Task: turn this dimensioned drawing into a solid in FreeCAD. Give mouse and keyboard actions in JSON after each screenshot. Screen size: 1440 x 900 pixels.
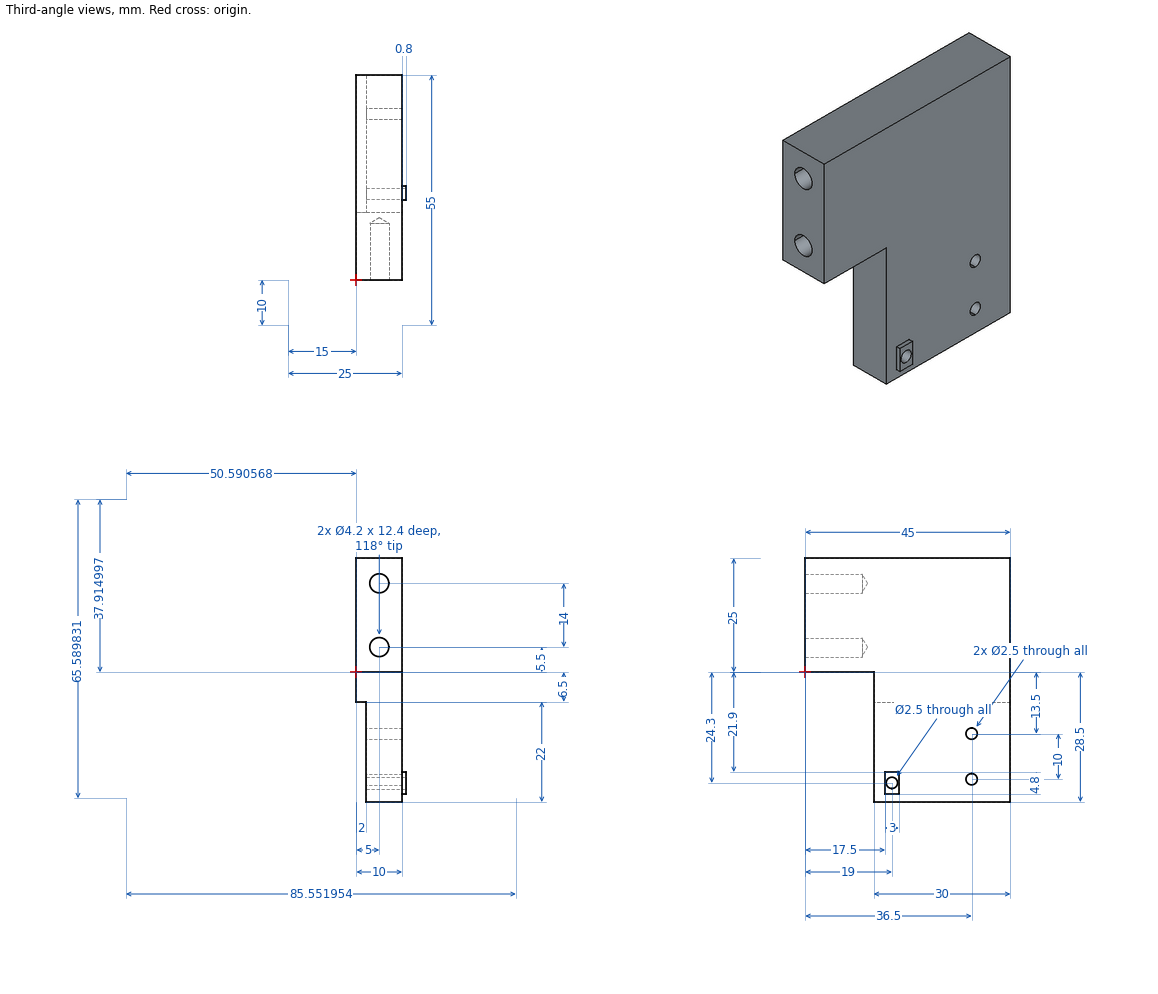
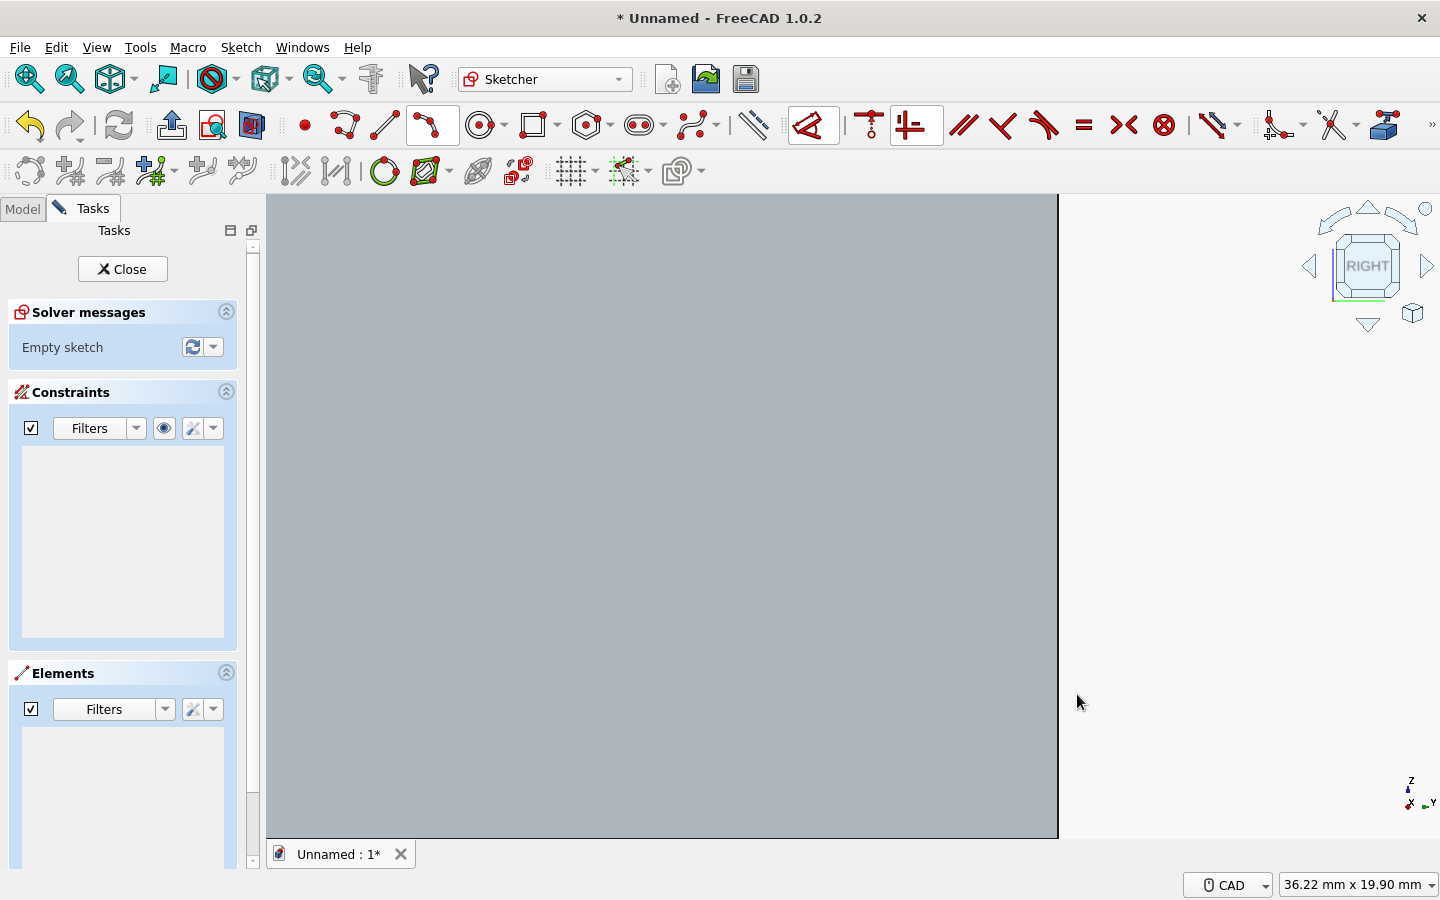
{"action": "left_click", "coordinate": [480, 126]}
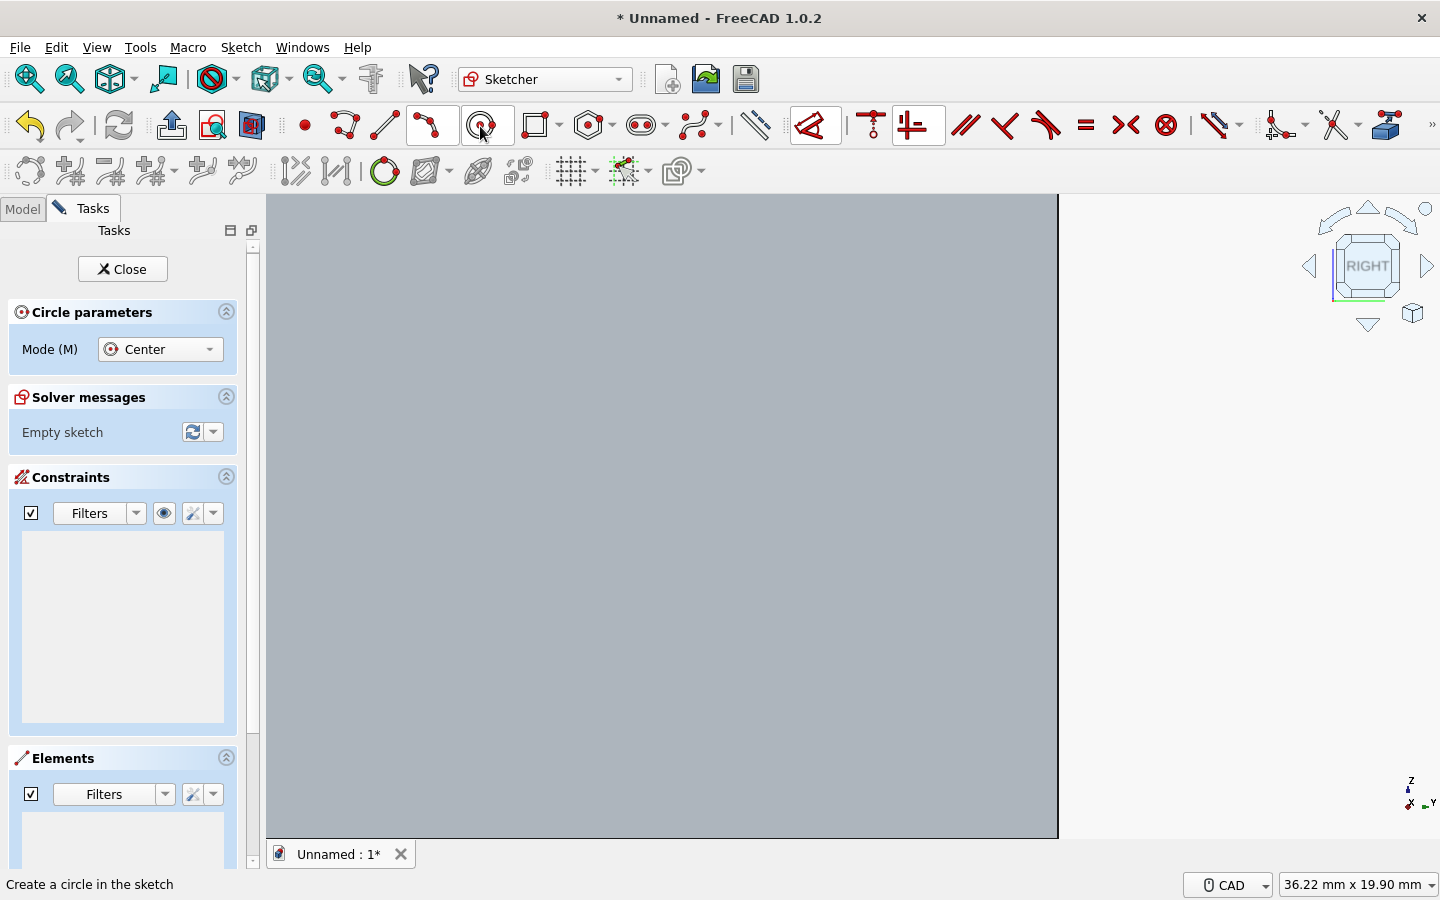
{"action": "left_click", "coordinate": [782, 353]}
{"action": "left_click", "coordinate": [811, 324]}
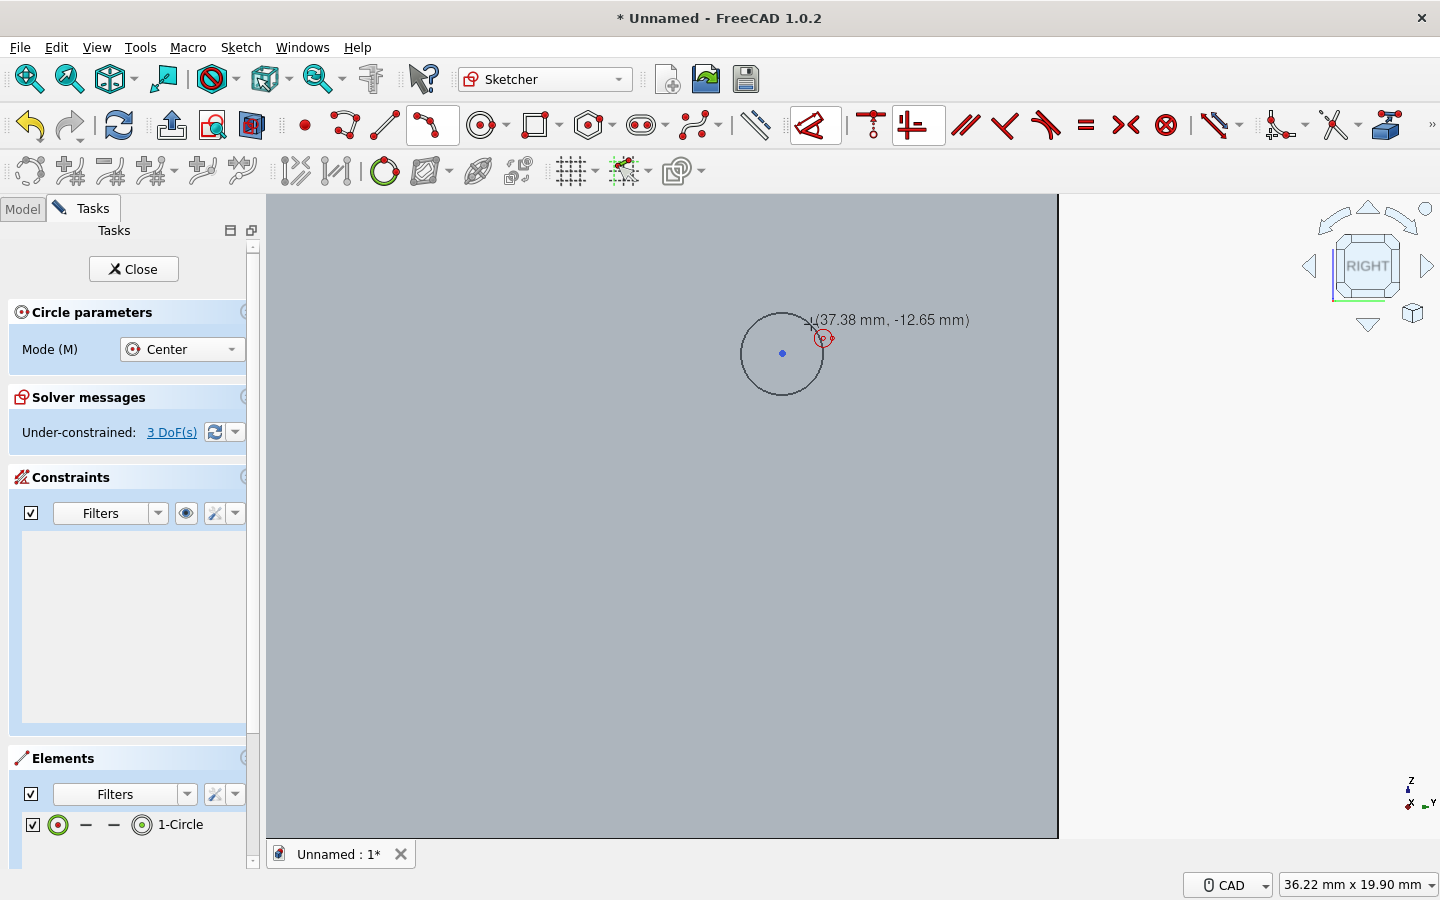
{"action": "left_click", "coordinate": [782, 677]}
{"action": "left_click", "coordinate": [811, 648]}
{"action": "key", "text": "Escape"}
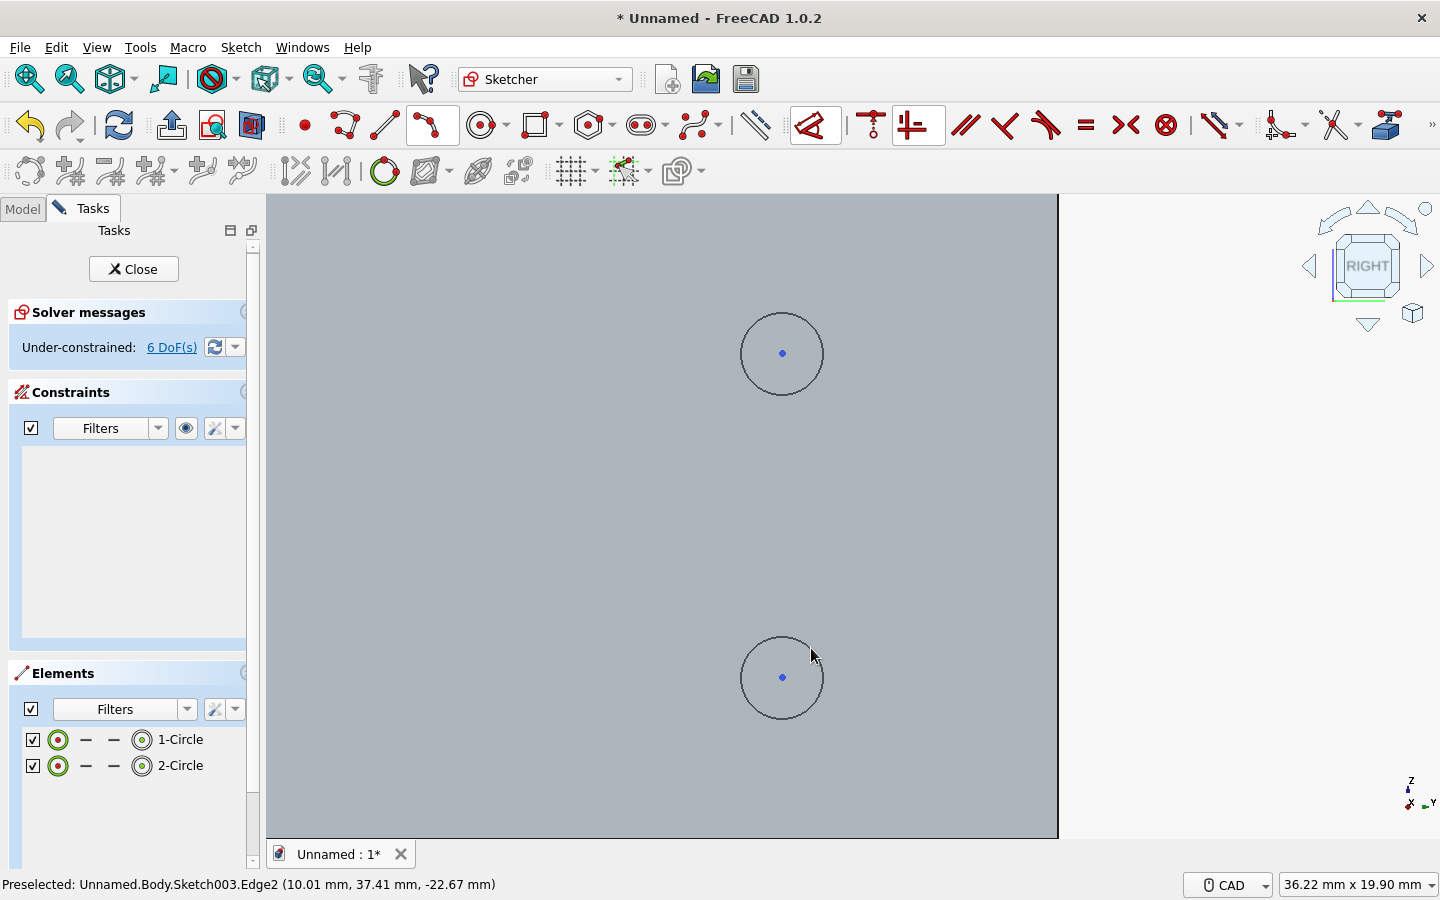
{"action": "left_click", "coordinate": [811, 325]}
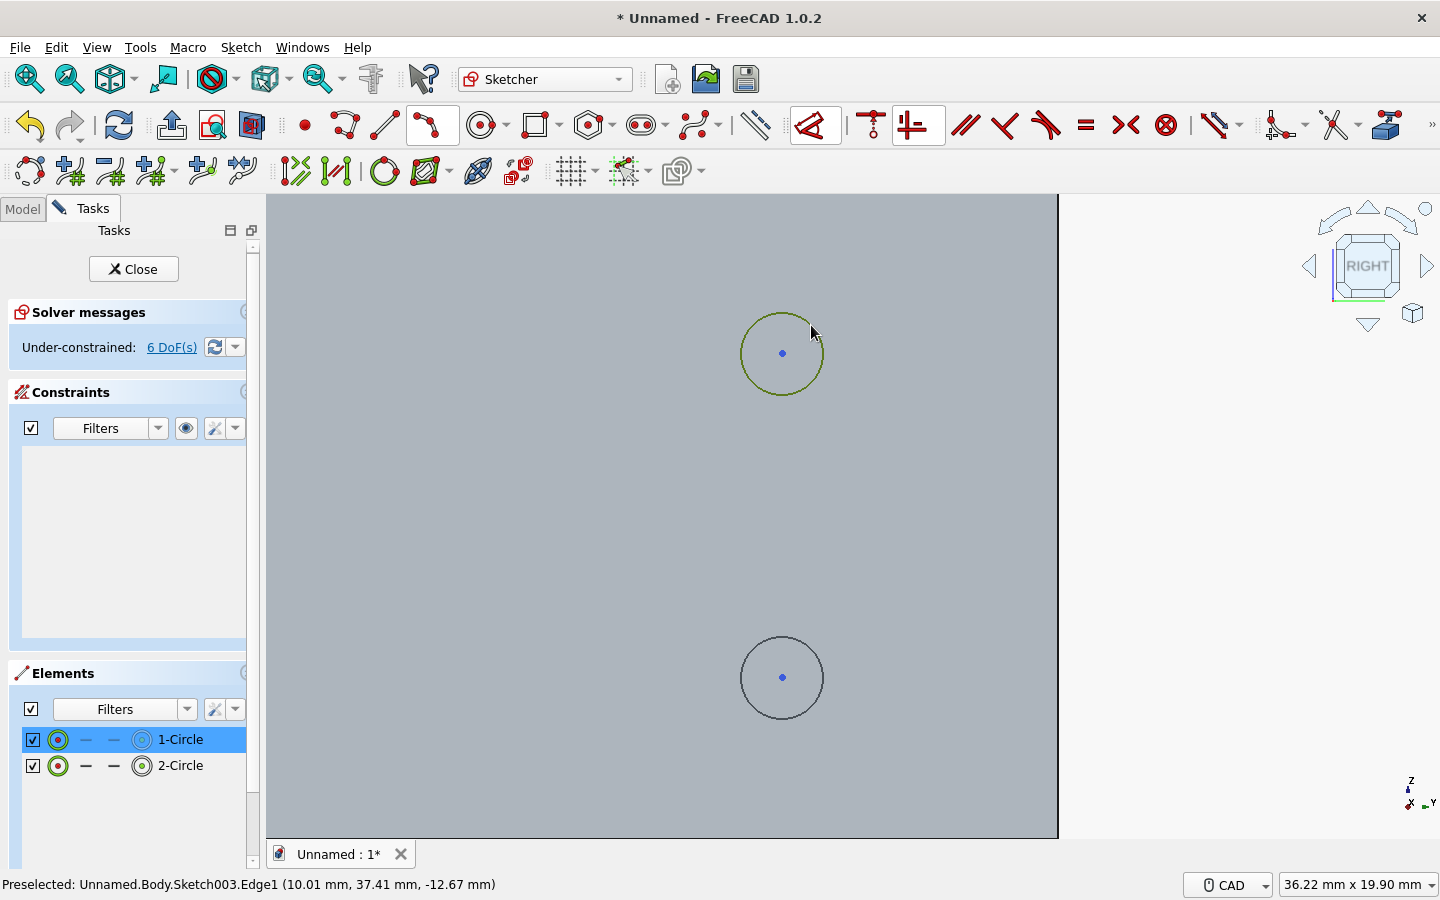
{"action": "left_click", "coordinate": [811, 649]}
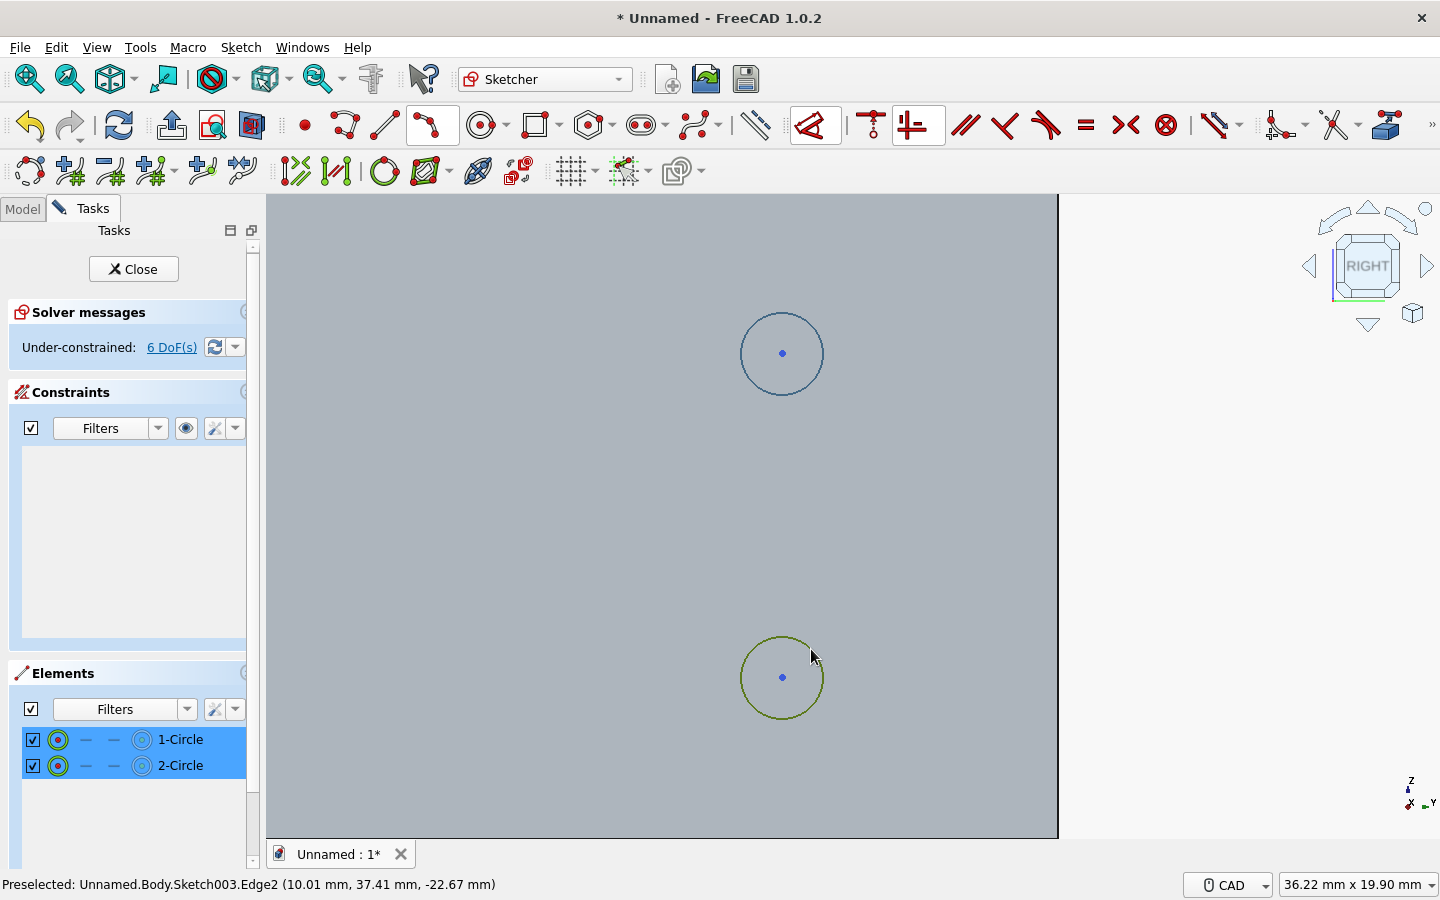
{"action": "key", "text": "e"}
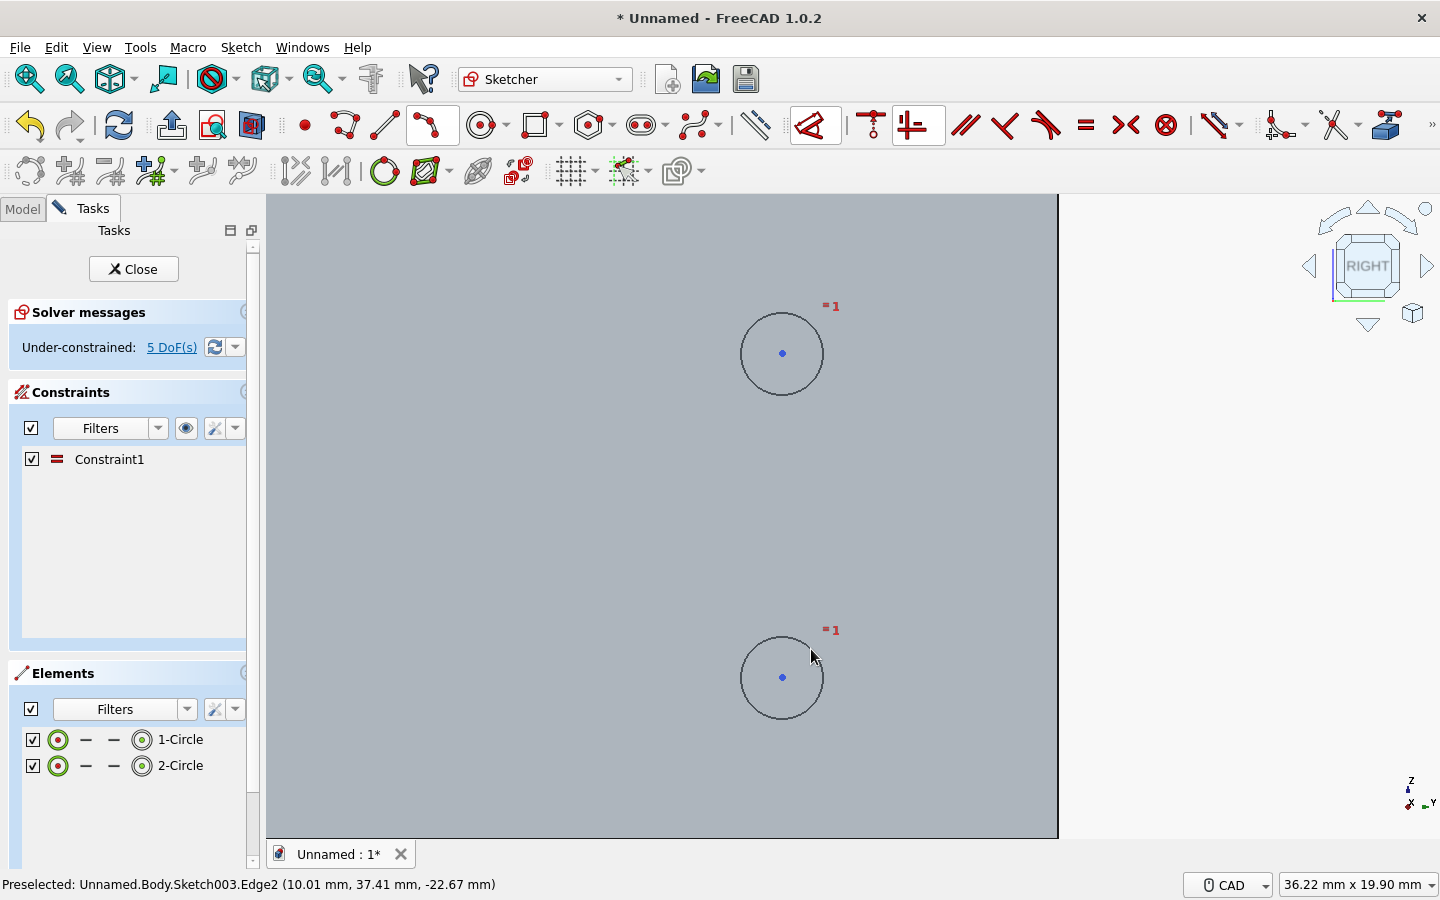
{"action": "left_click", "coordinate": [782, 354]}